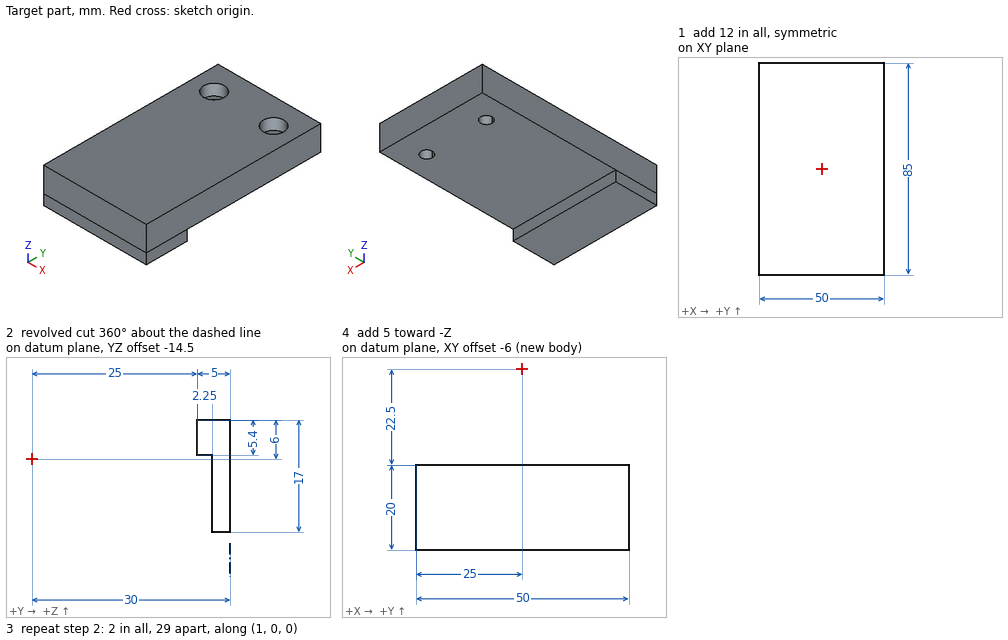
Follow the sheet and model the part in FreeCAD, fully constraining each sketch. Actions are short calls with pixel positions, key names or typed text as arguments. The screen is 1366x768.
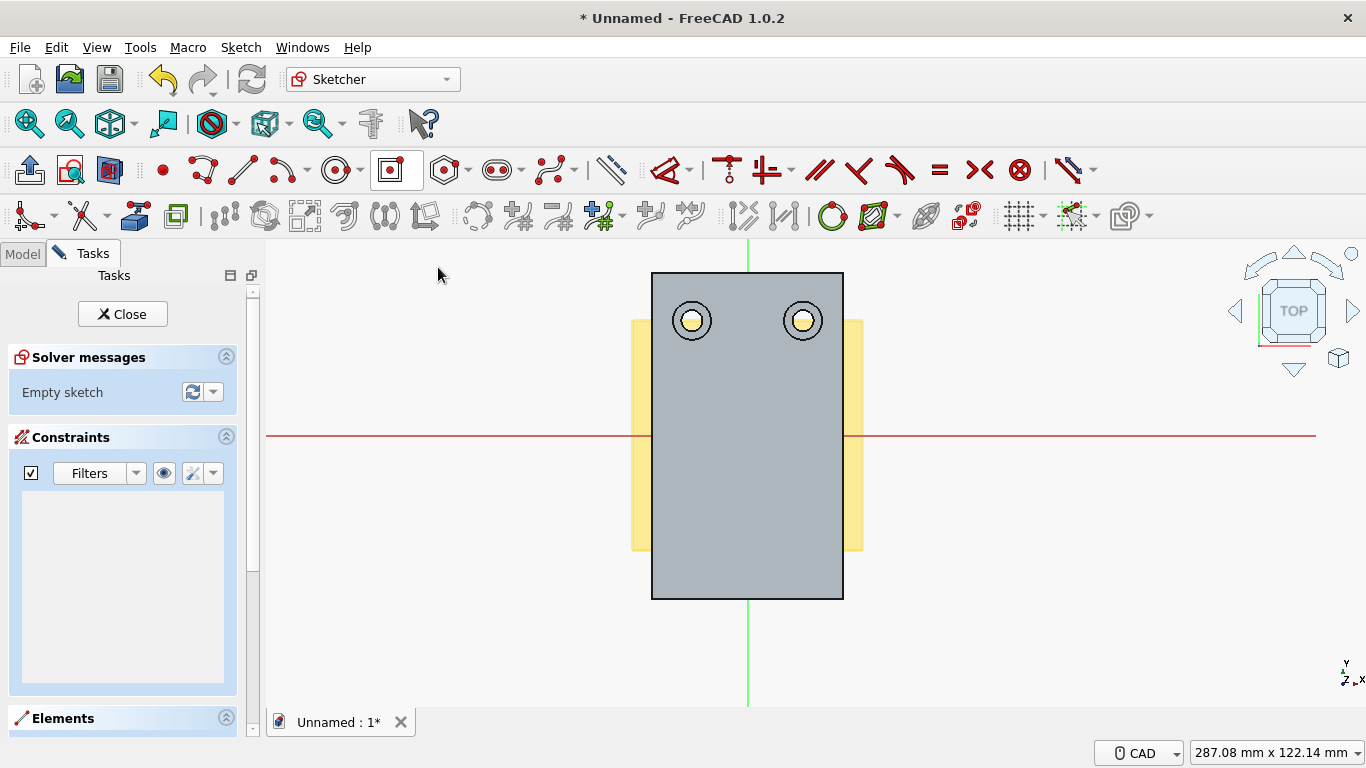
scroll(748, 571, up, 3)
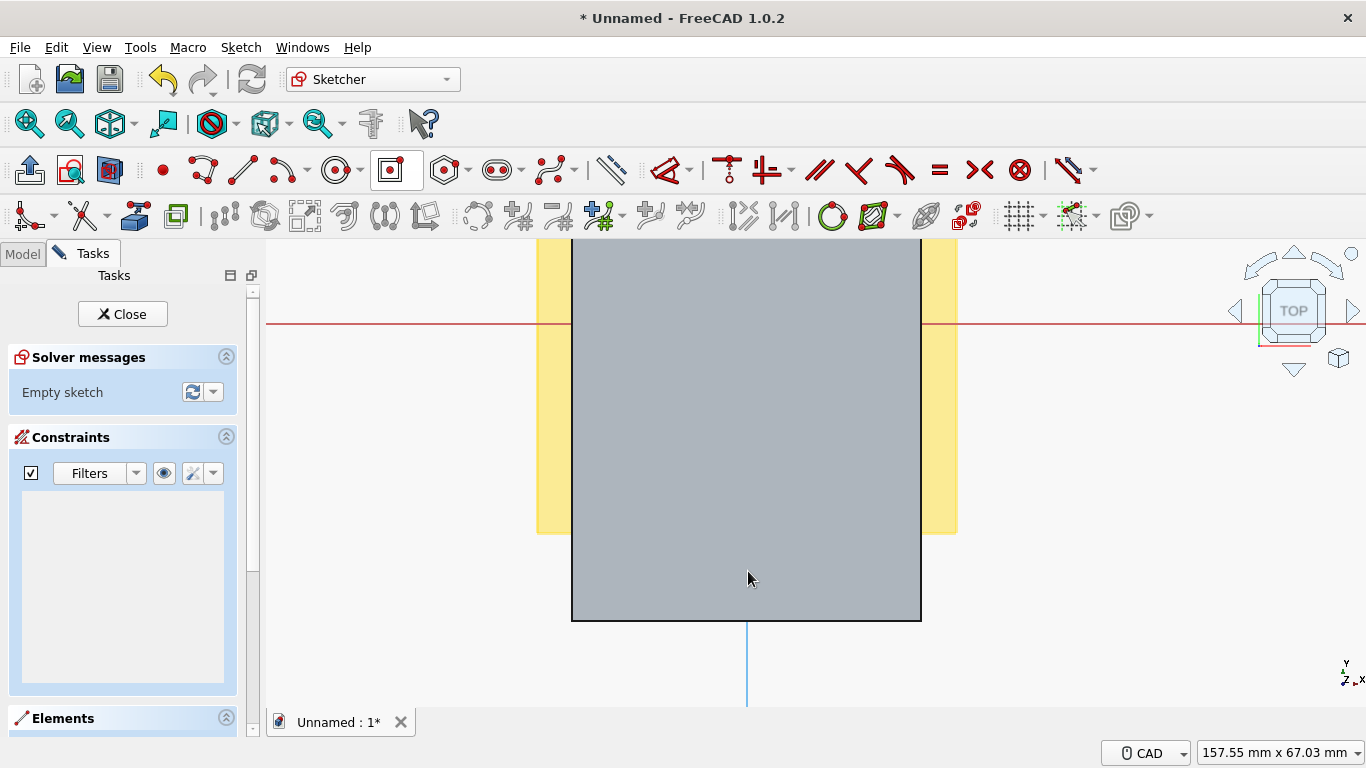
click(418, 170)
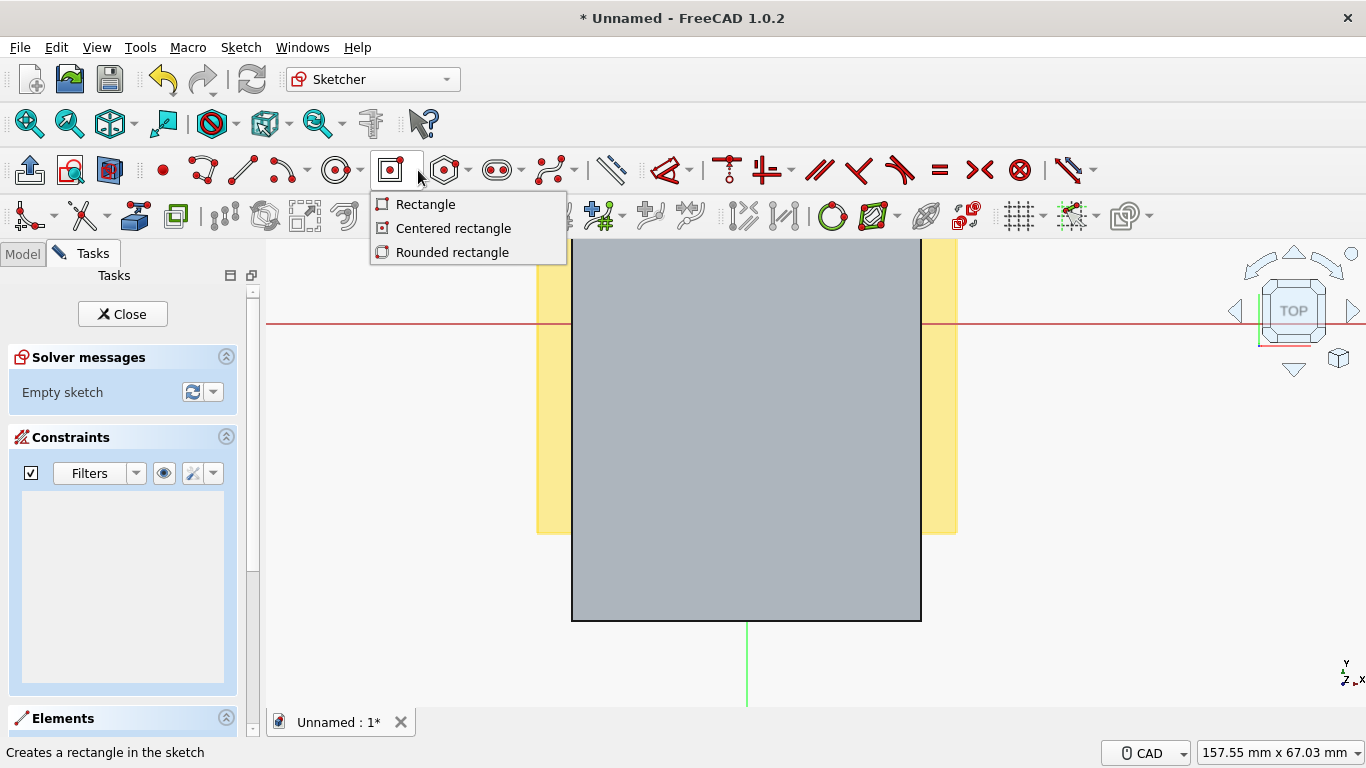
click(468, 204)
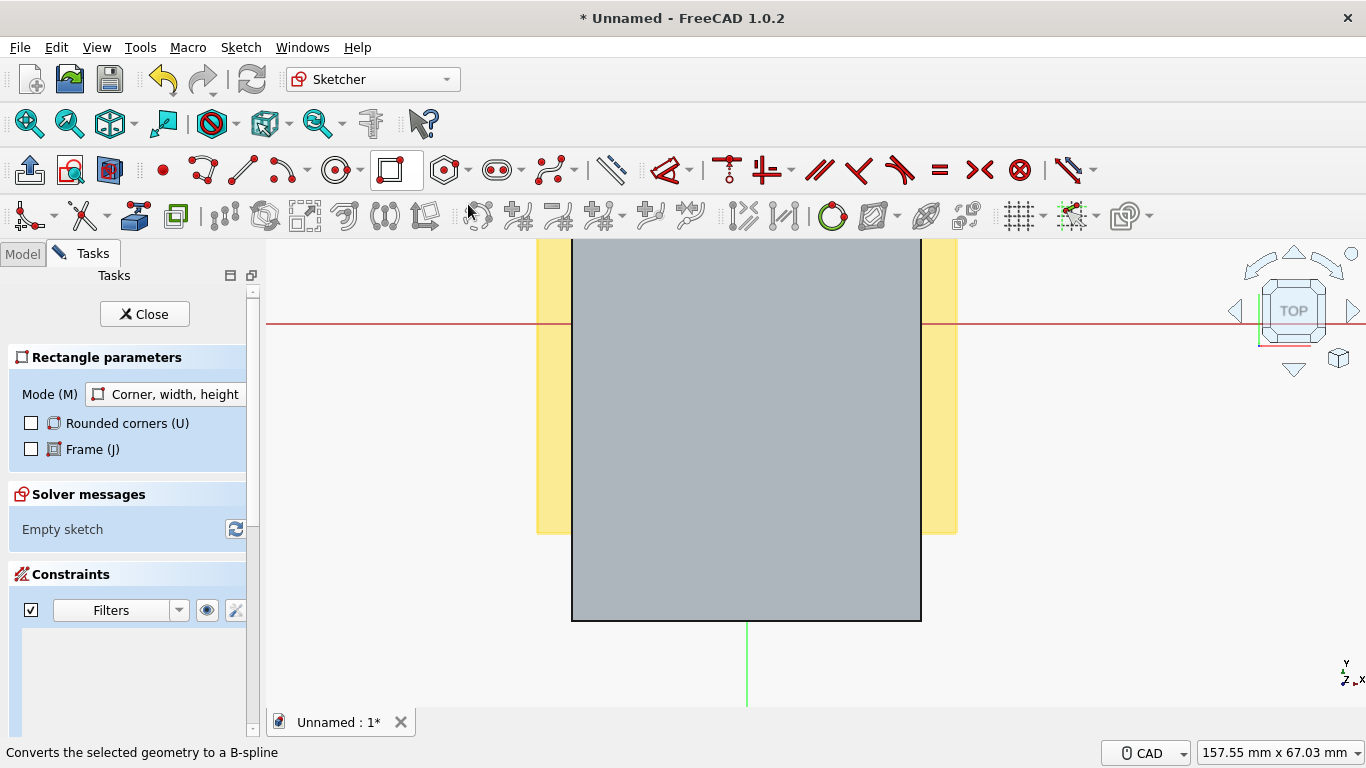
click(572, 481)
click(921, 621)
key(Escape)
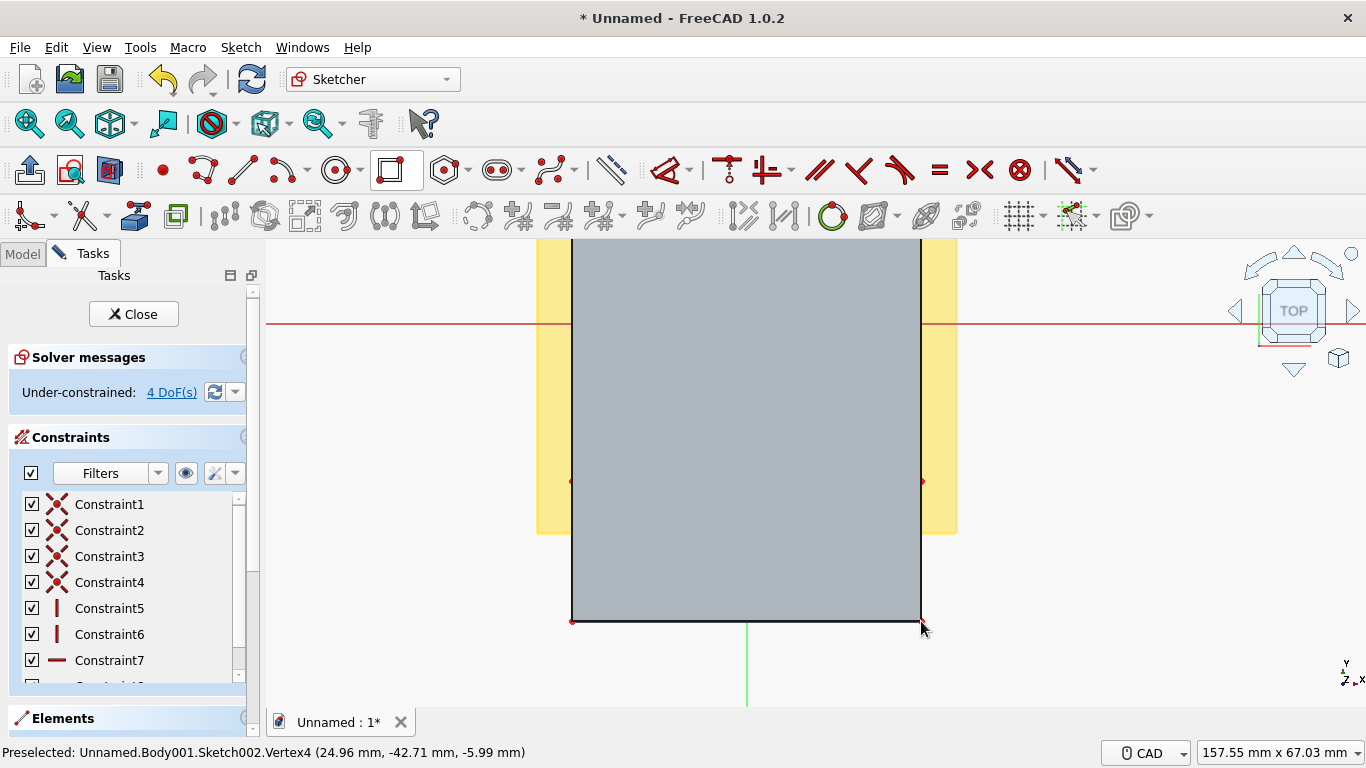
key(d)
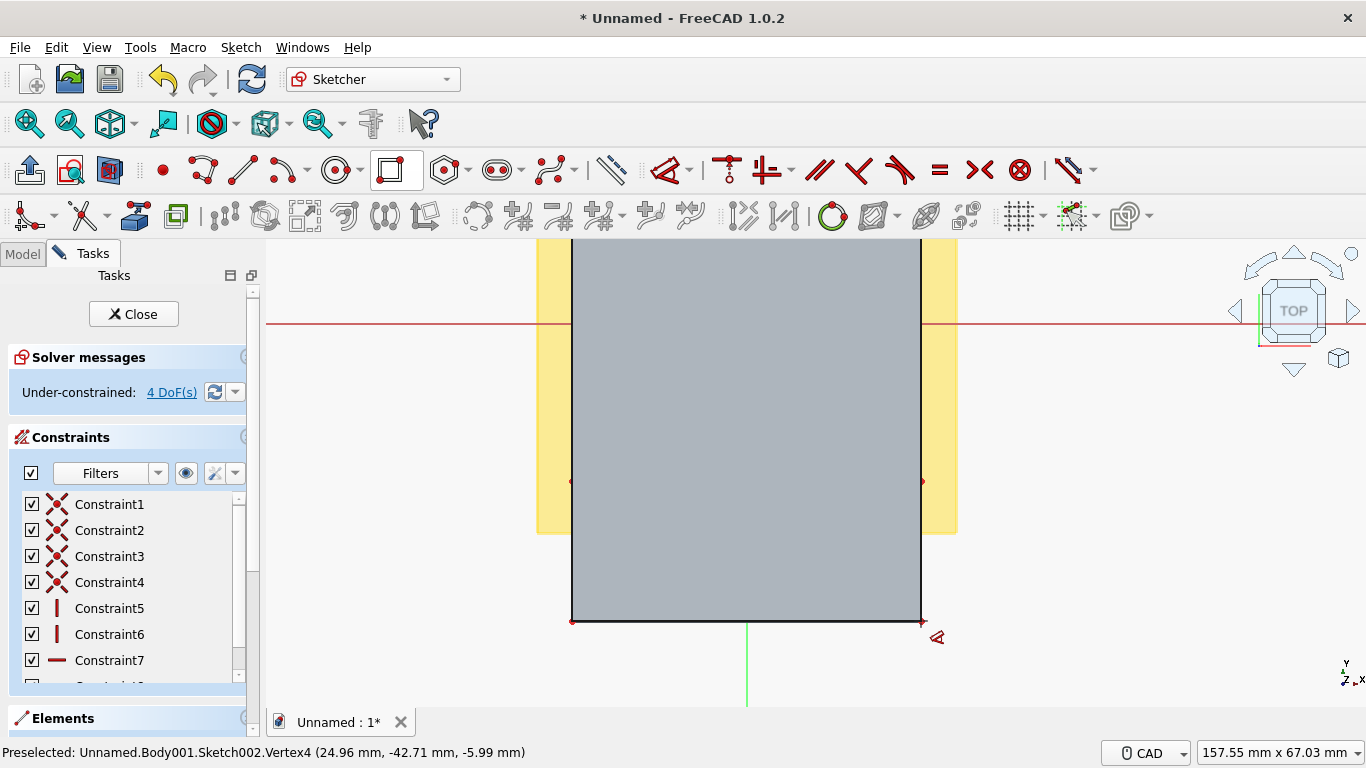
click(572, 524)
click(538, 552)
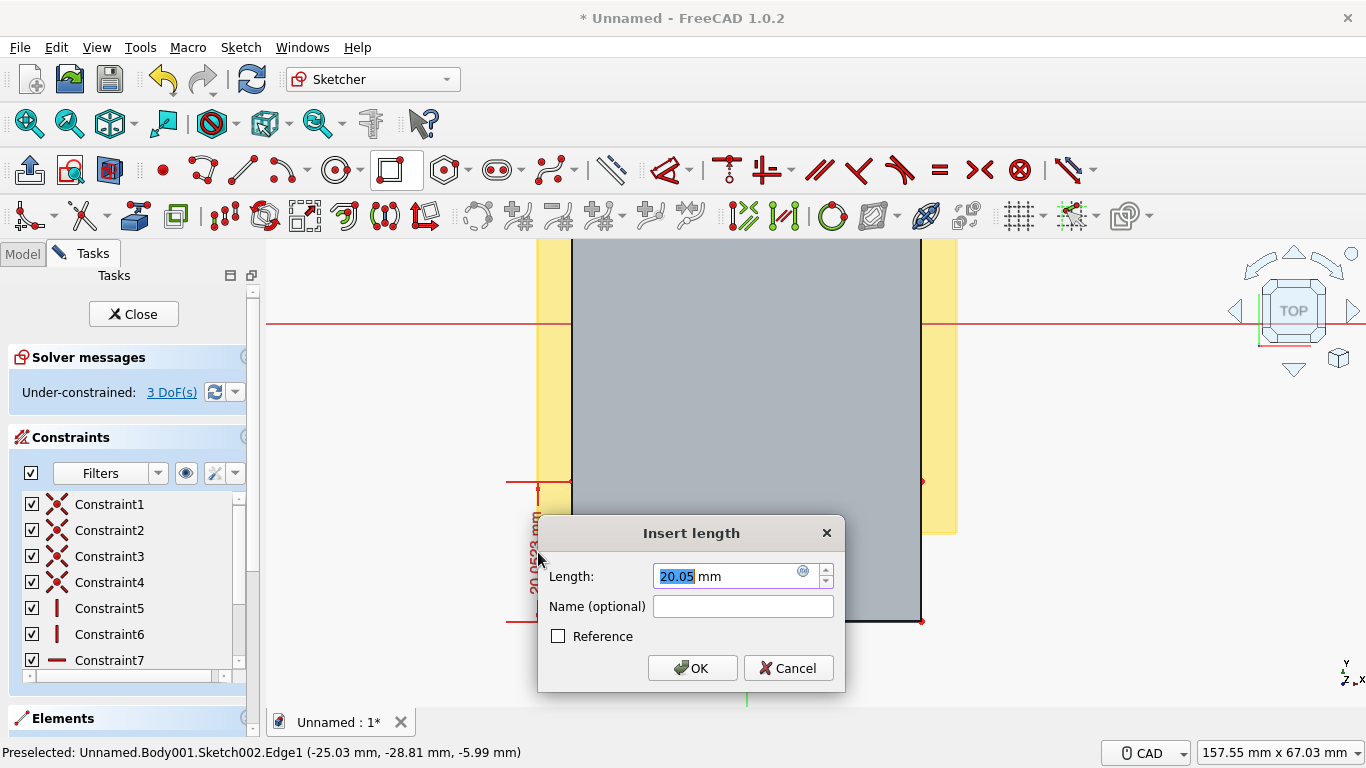
text(20)
key(Return)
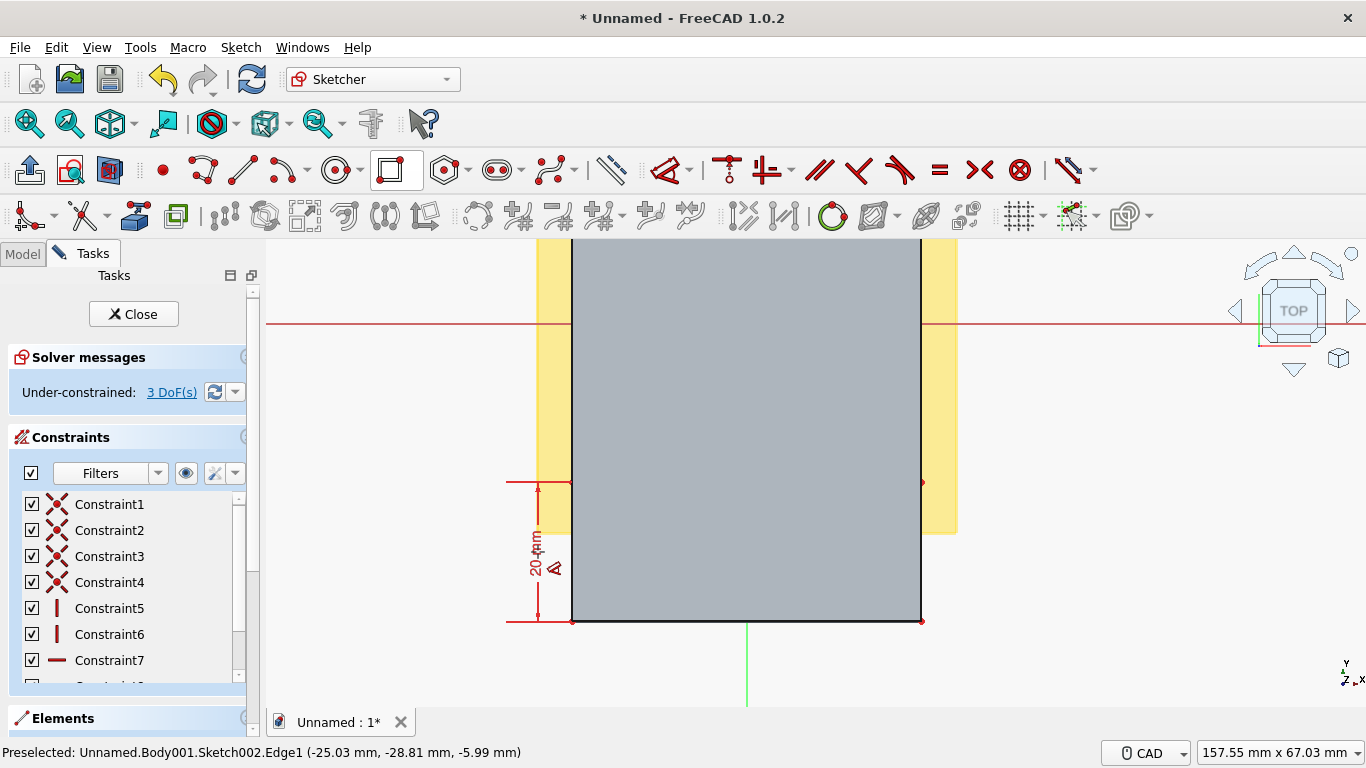
click(677, 622)
click(666, 656)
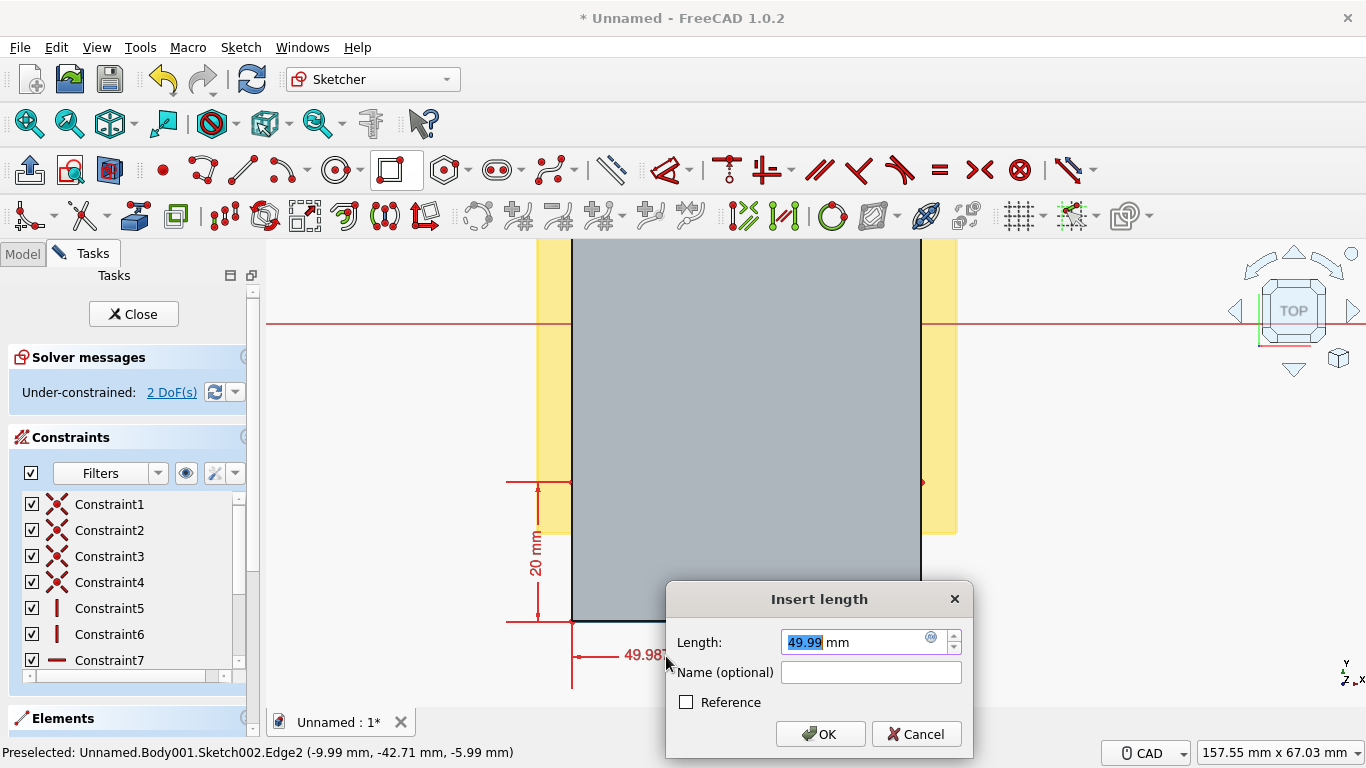
text(50)
key(Return)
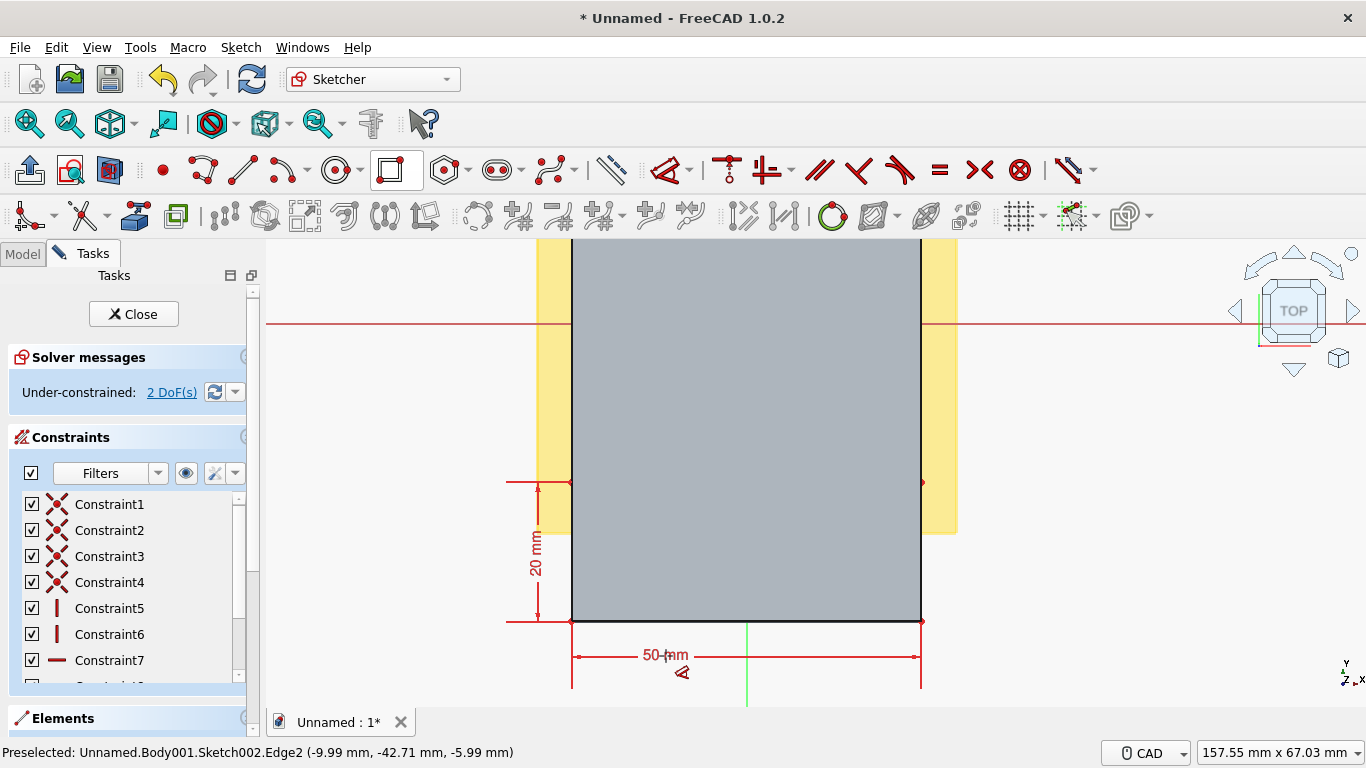
click(572, 482)
click(659, 290)